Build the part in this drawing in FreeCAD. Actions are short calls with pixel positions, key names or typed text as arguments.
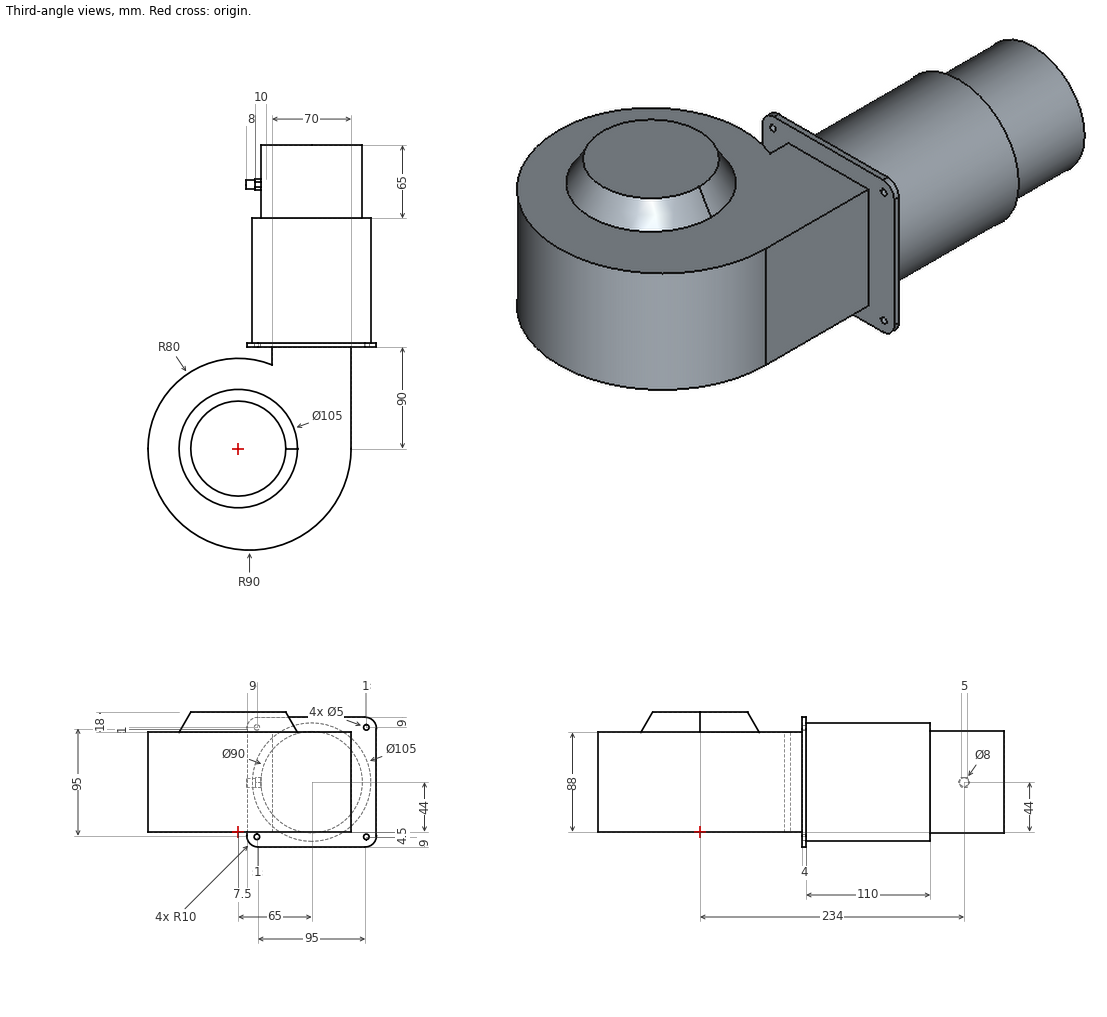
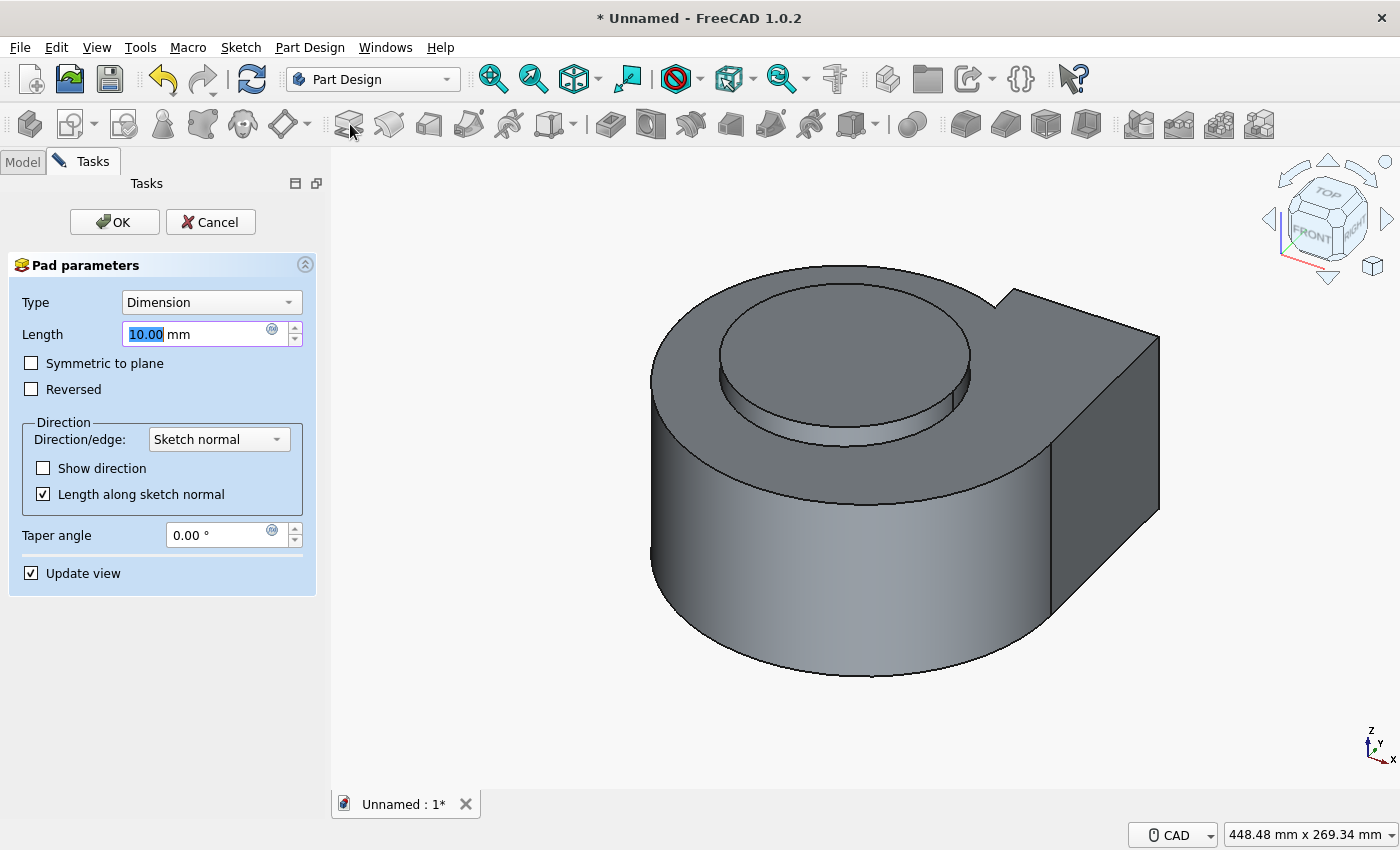
text(18)
key(Tab)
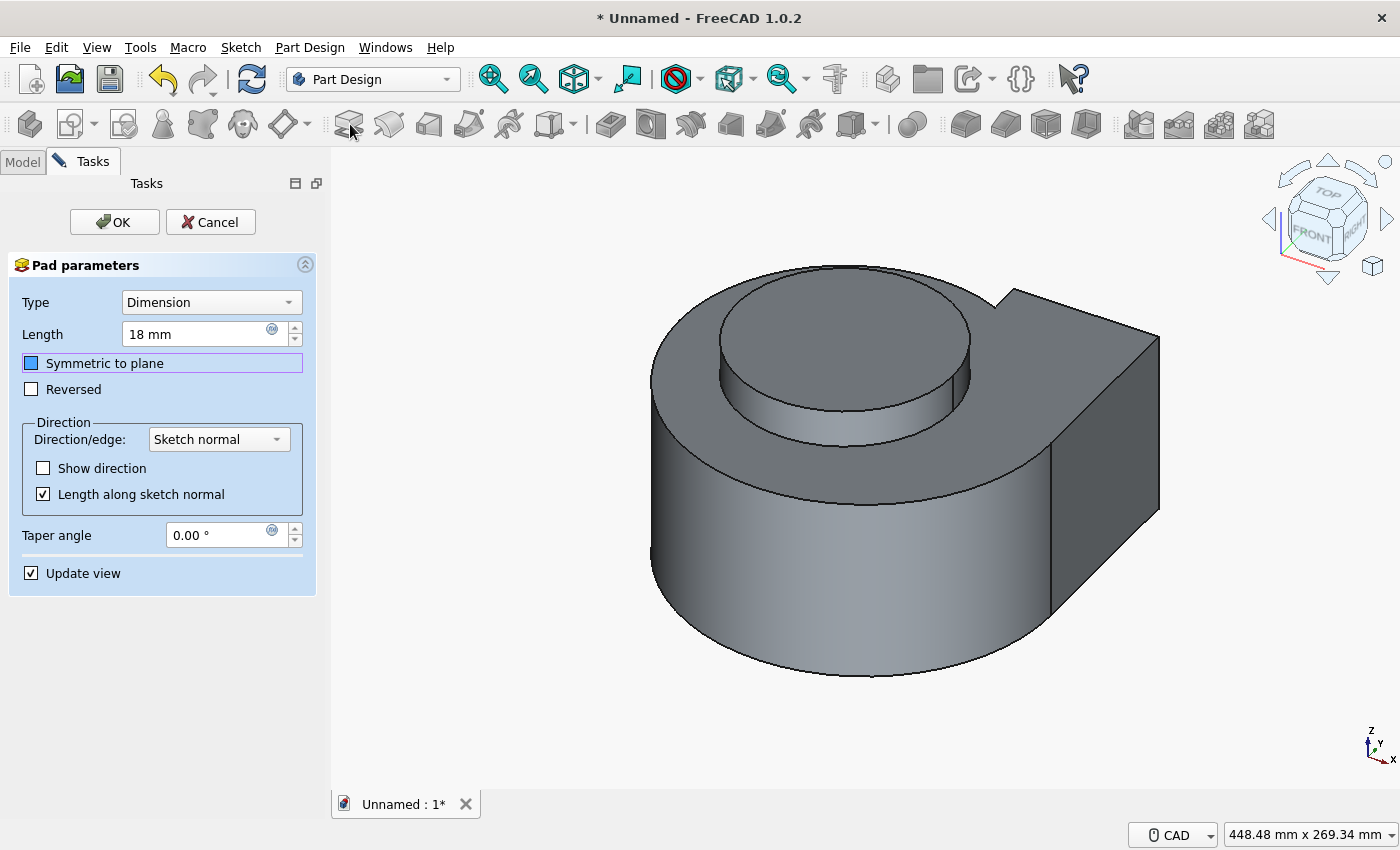
triple_click(226, 535)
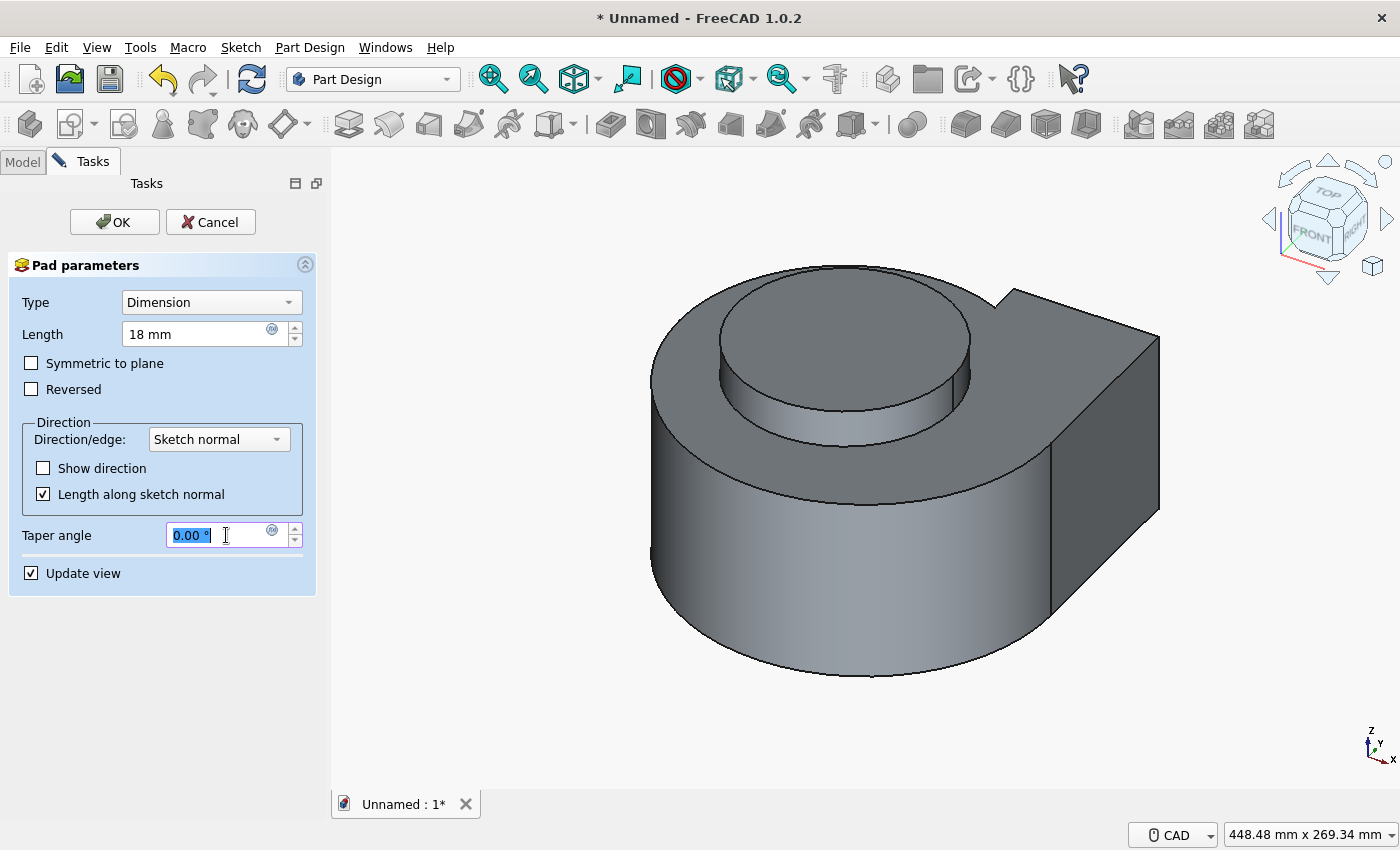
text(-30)
key(Tab)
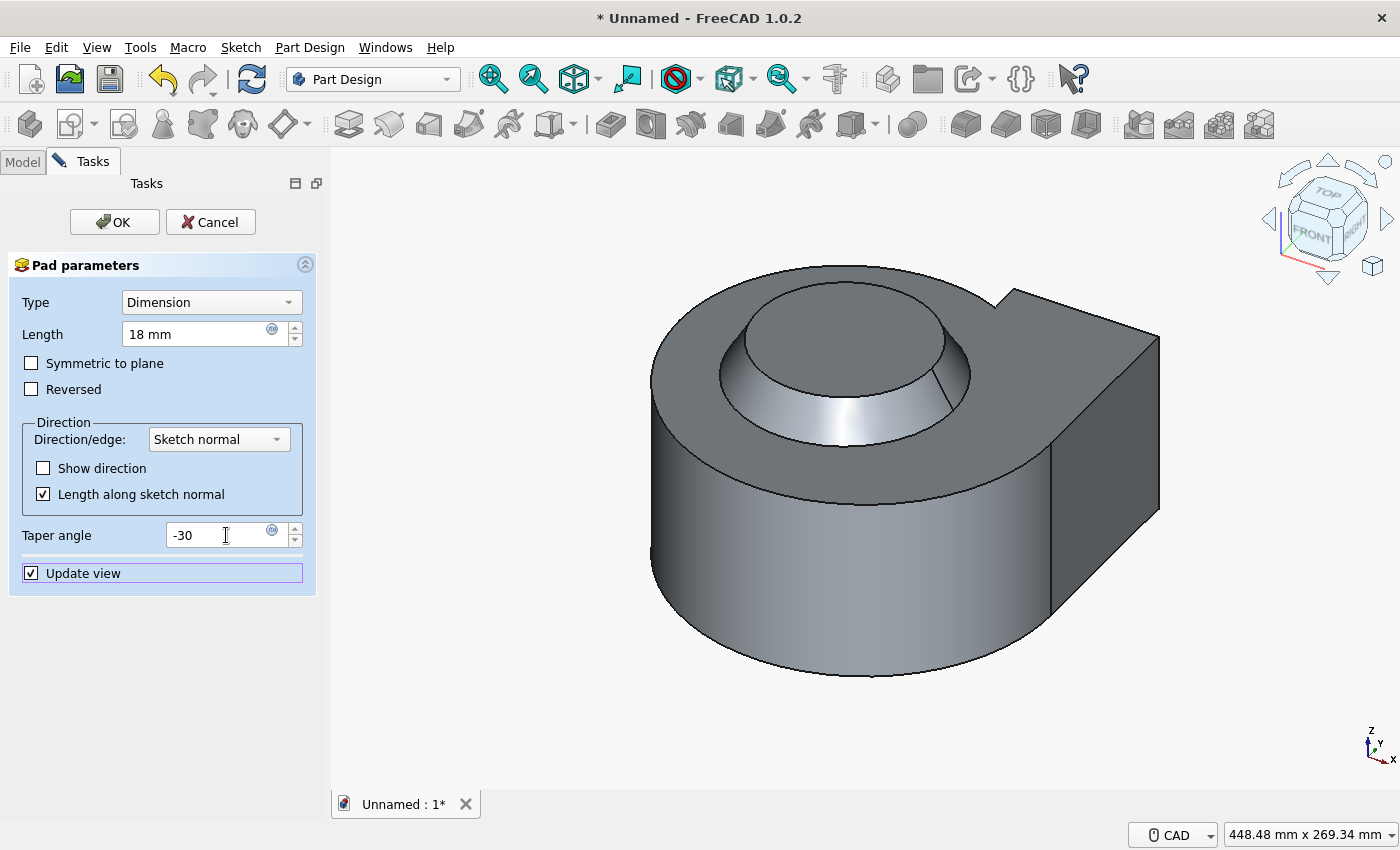
click(115, 222)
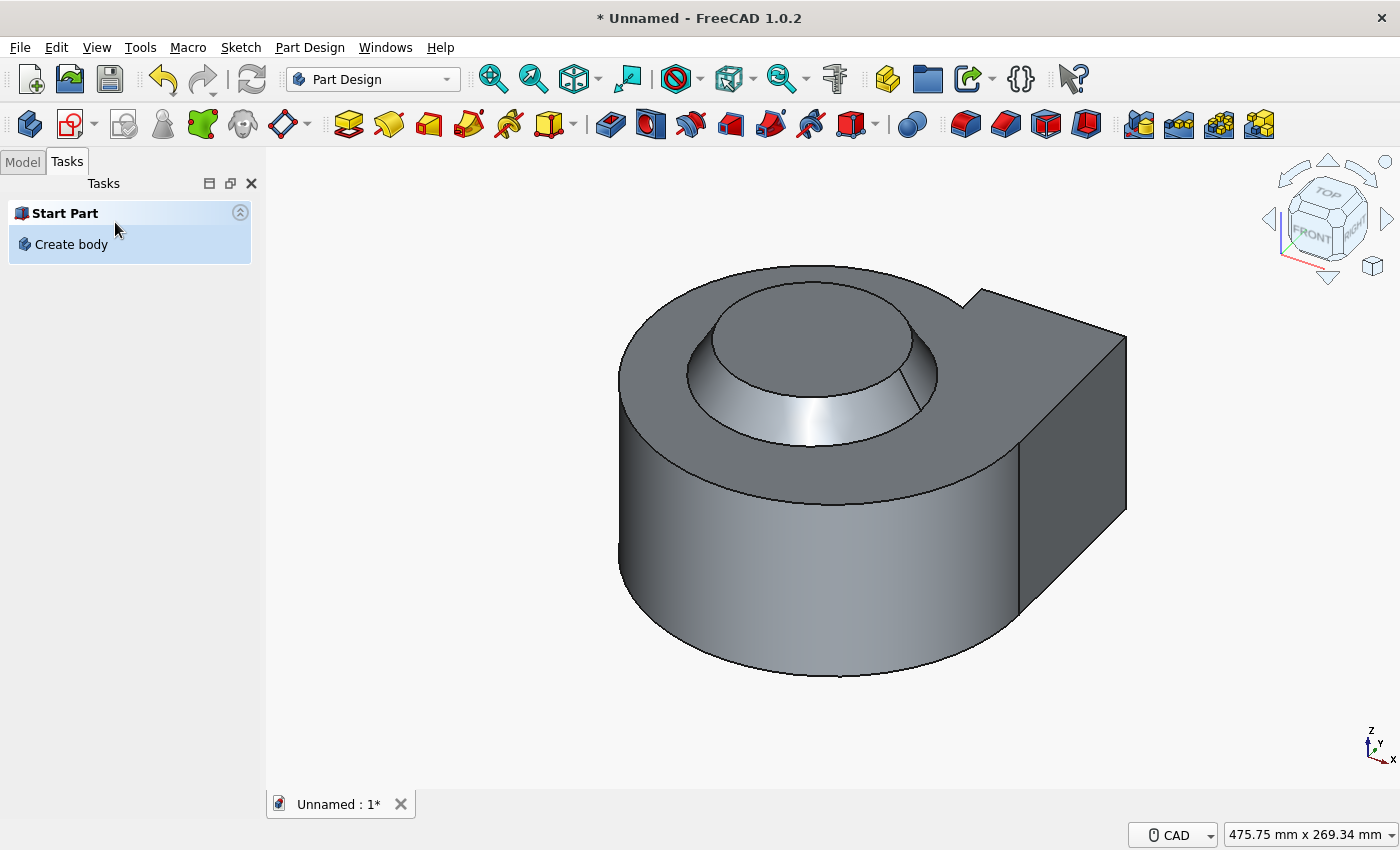
key(4)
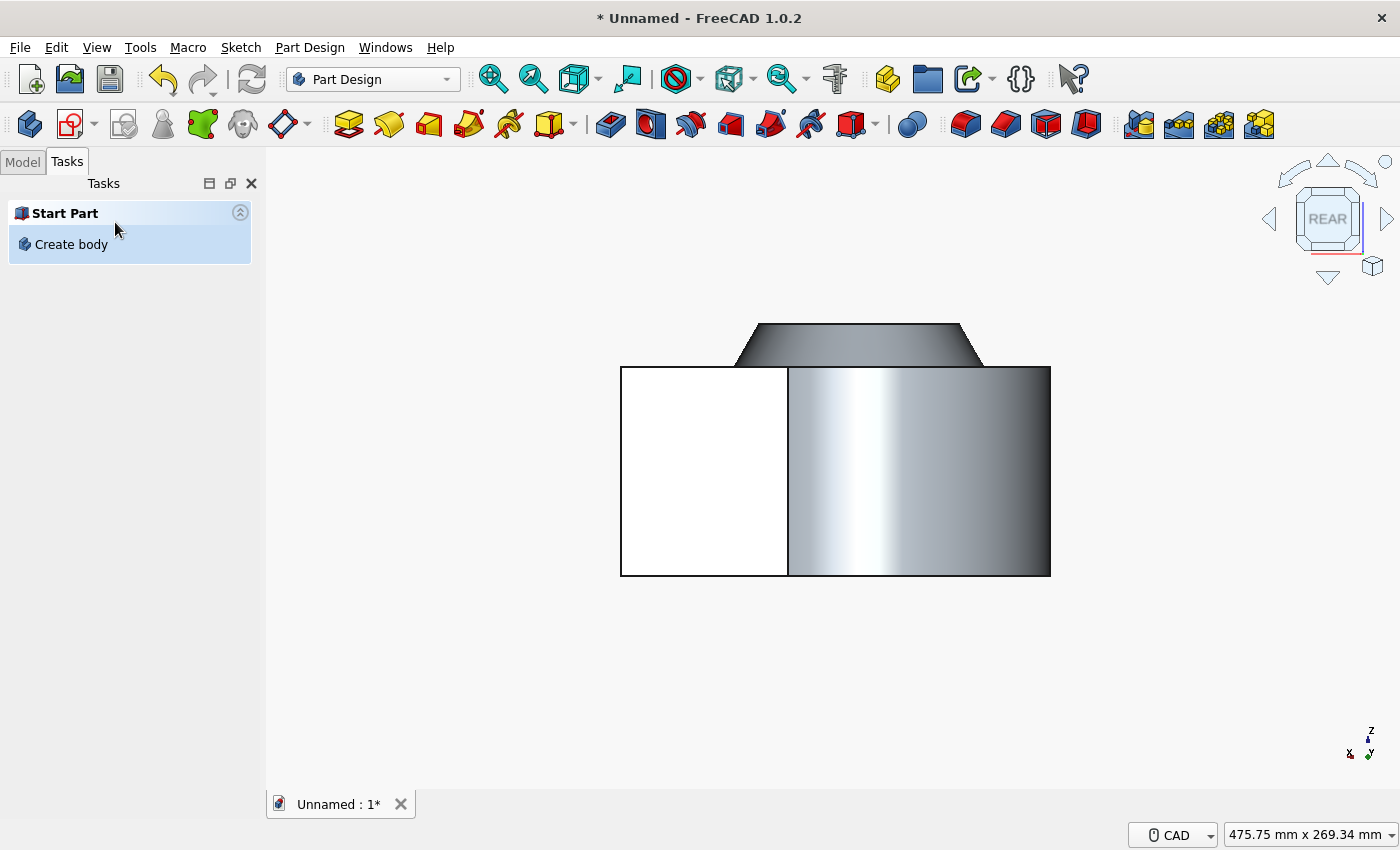
click(494, 80)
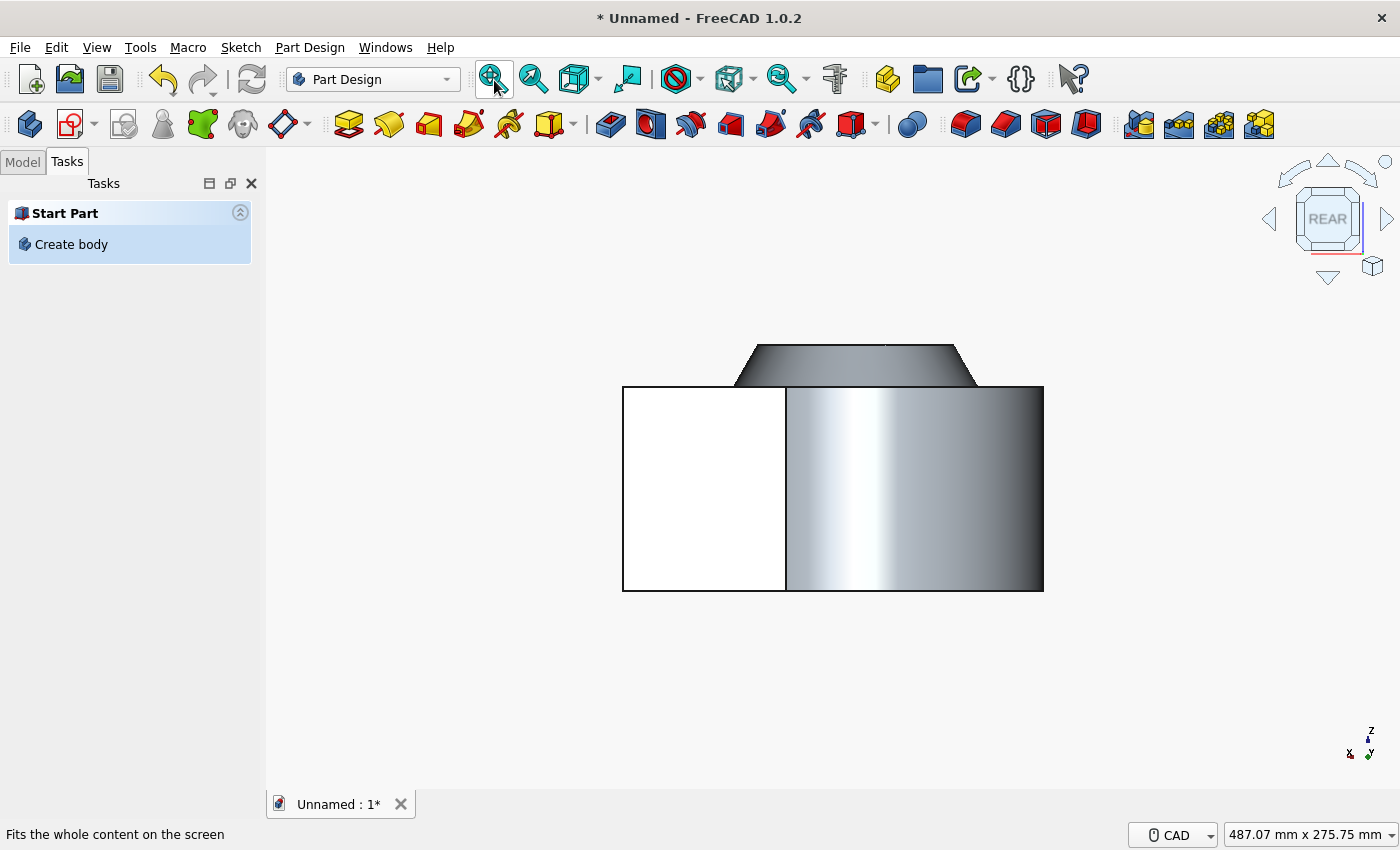
click(705, 488)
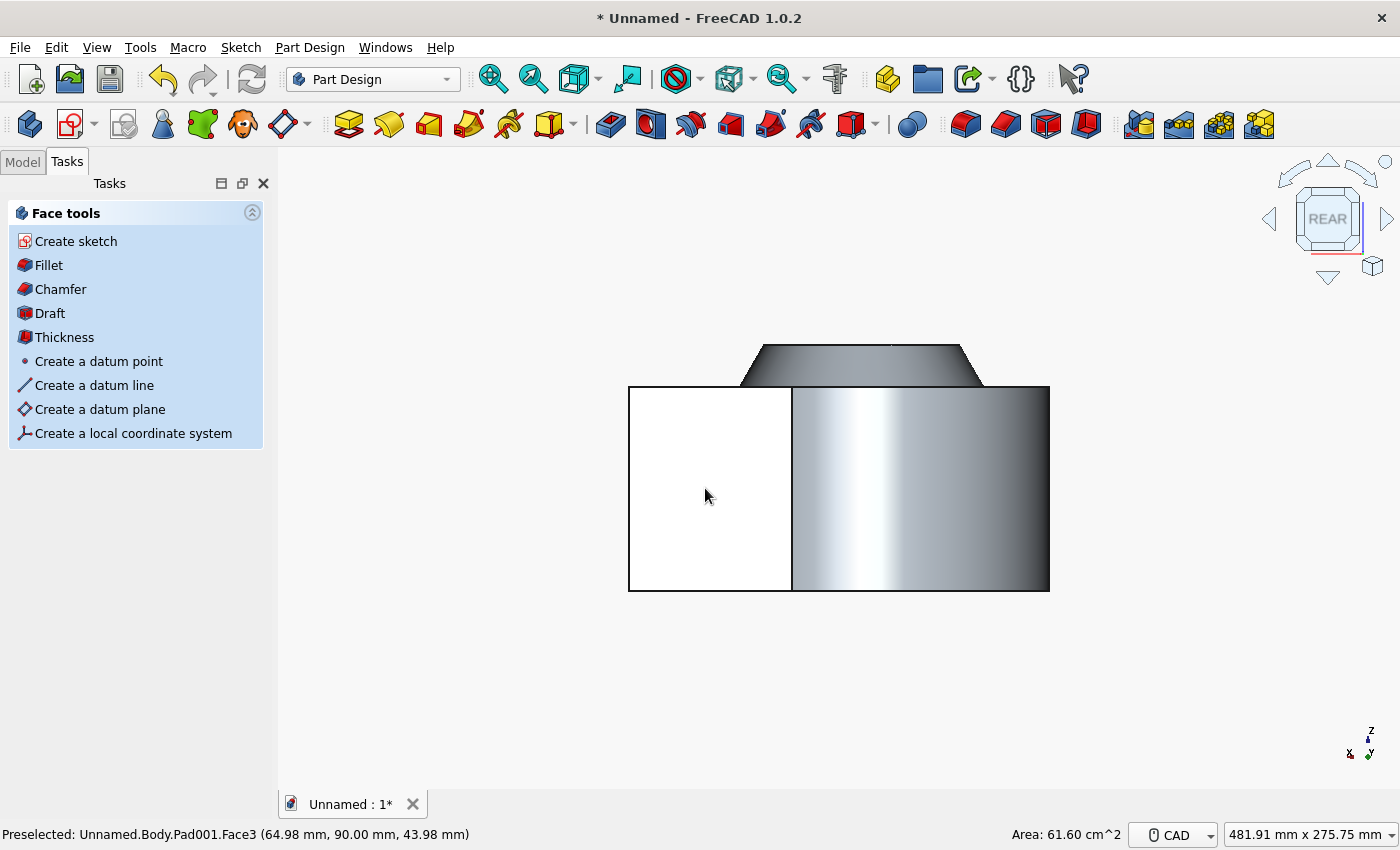
click(70, 124)